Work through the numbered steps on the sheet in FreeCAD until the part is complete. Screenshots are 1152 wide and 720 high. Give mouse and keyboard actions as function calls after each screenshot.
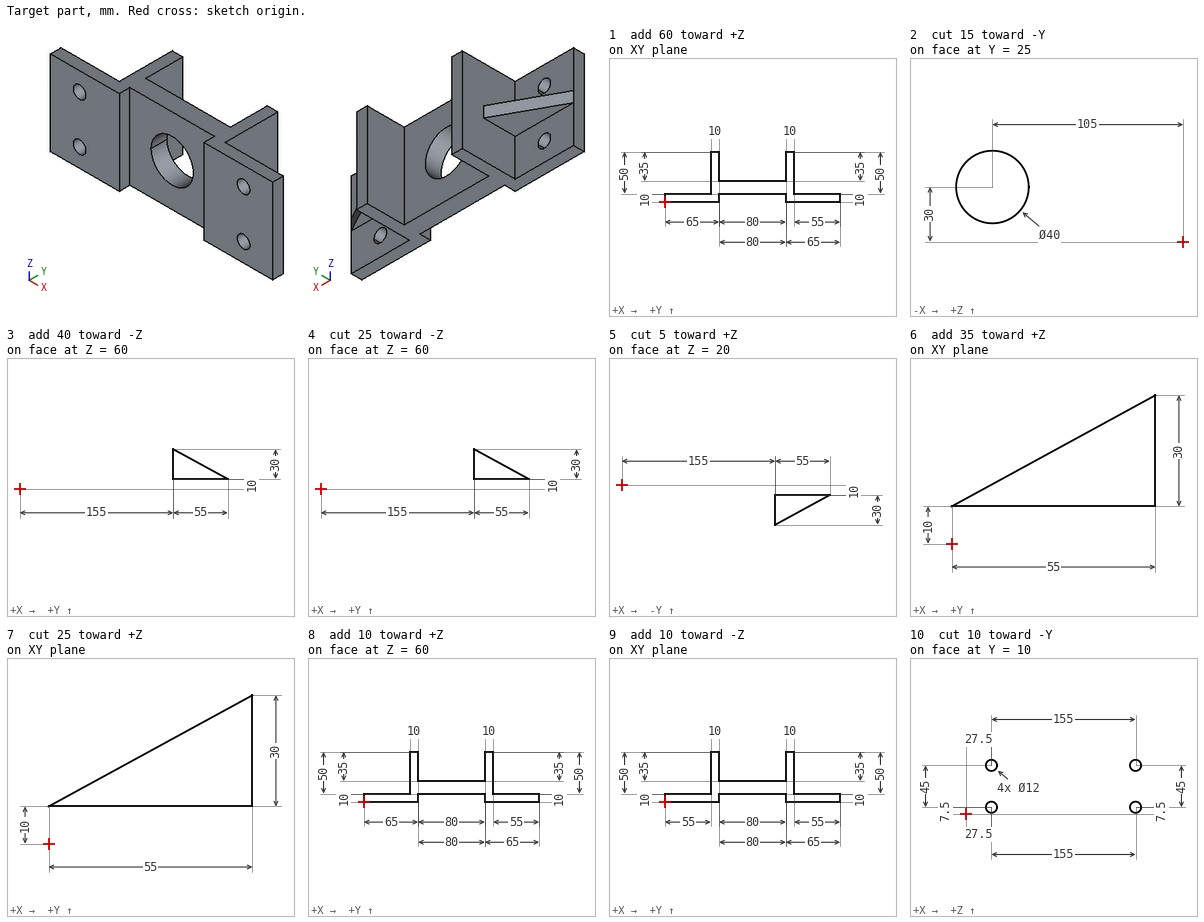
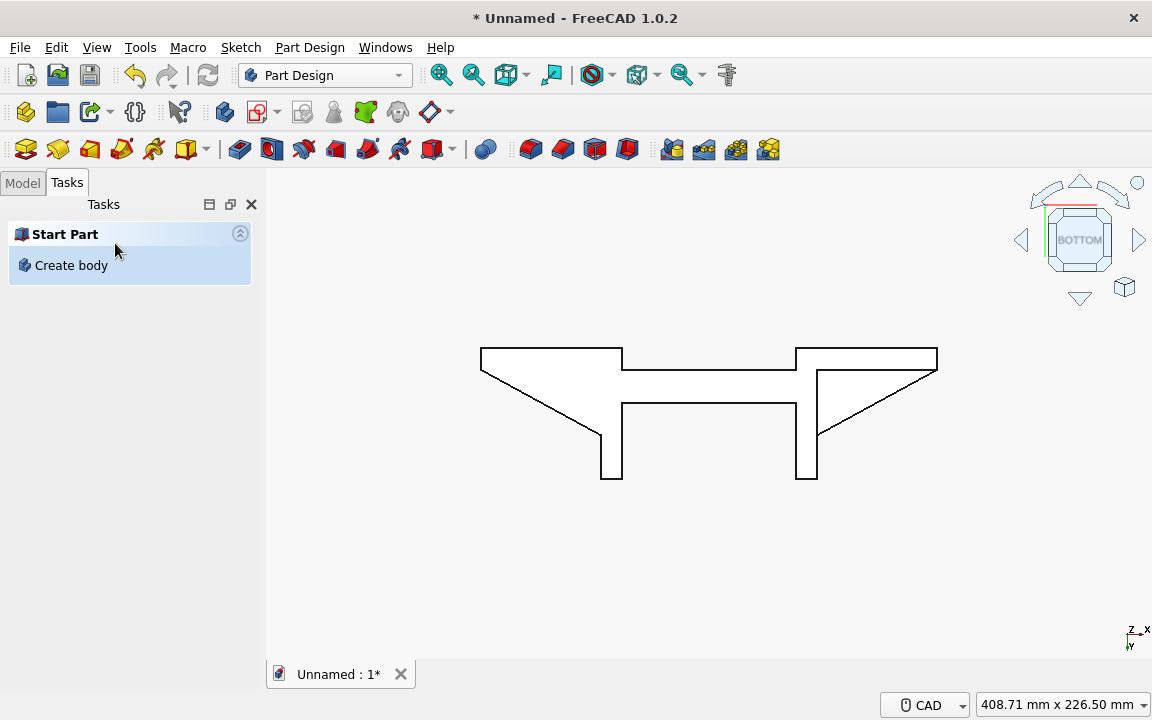
click(258, 112)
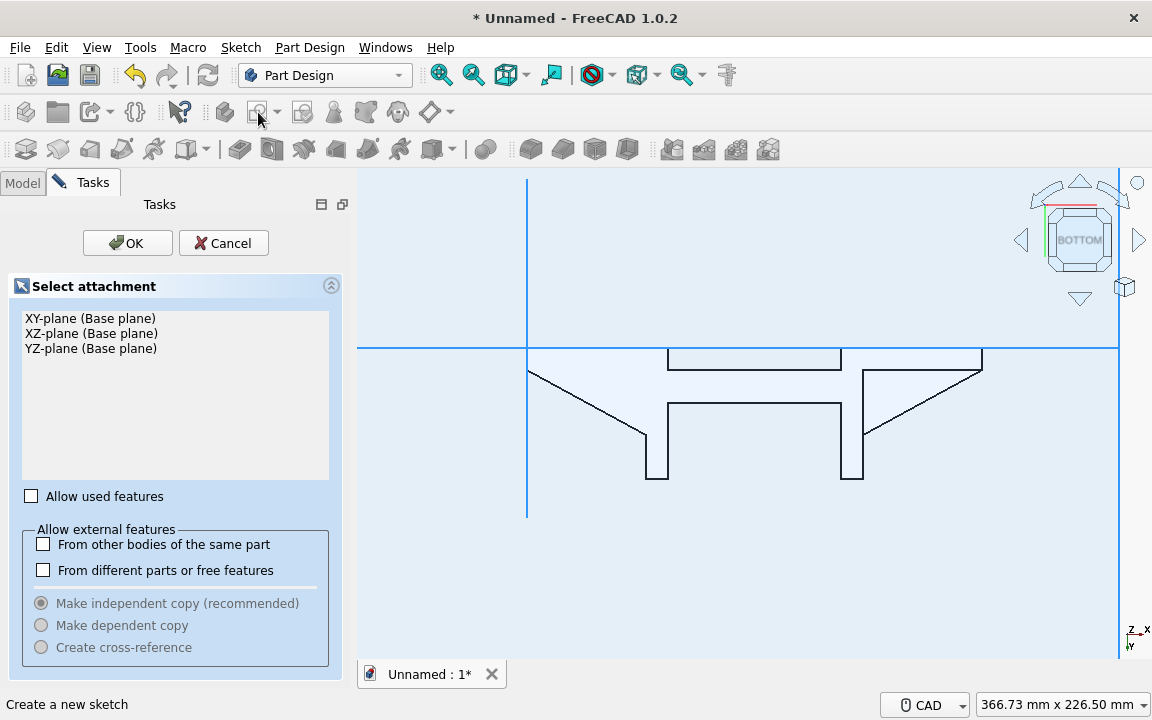
click(82, 318)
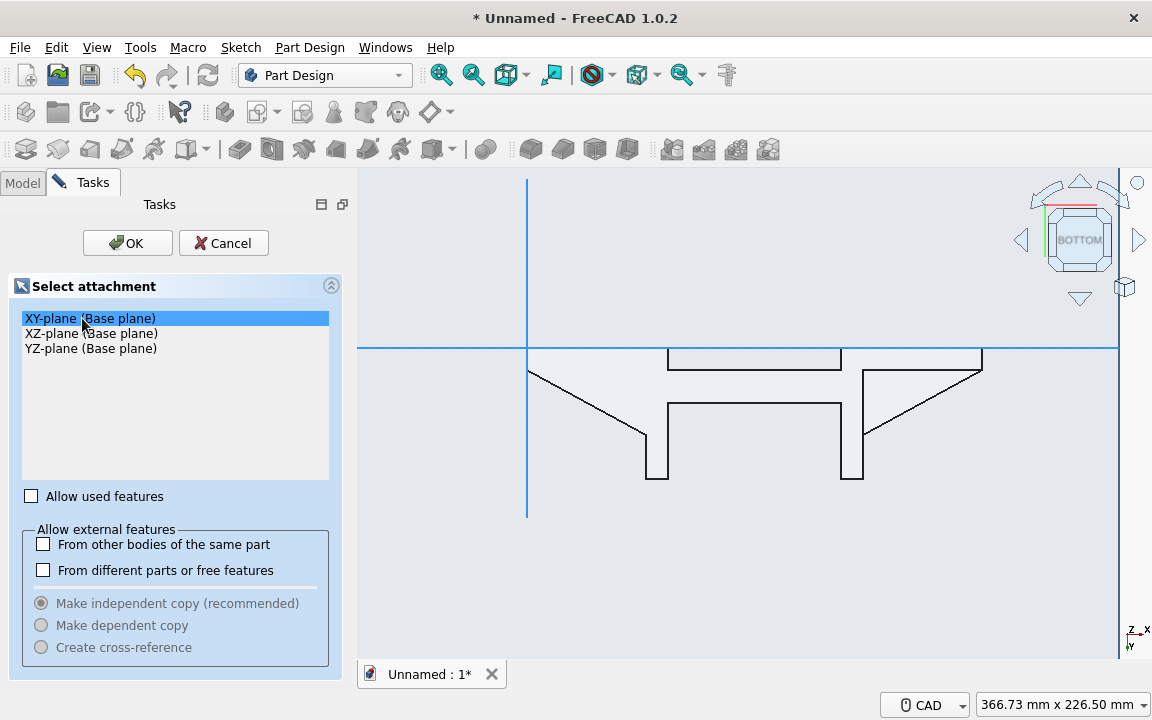
click(128, 243)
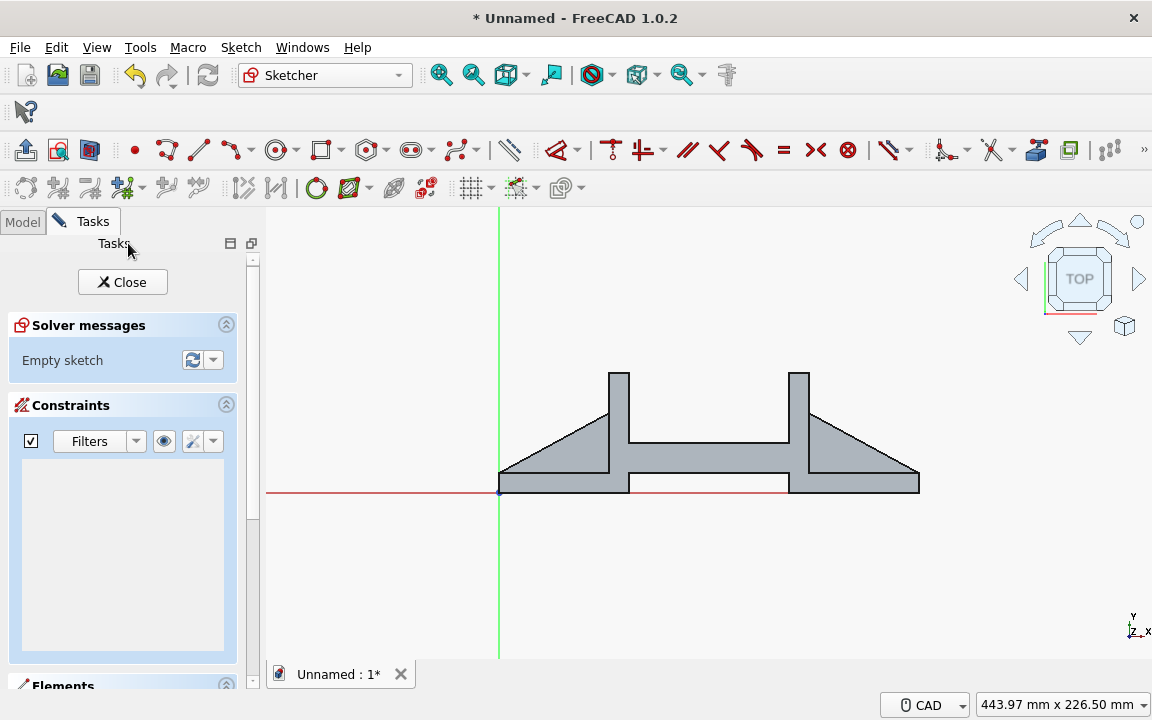
key(q)
key(s)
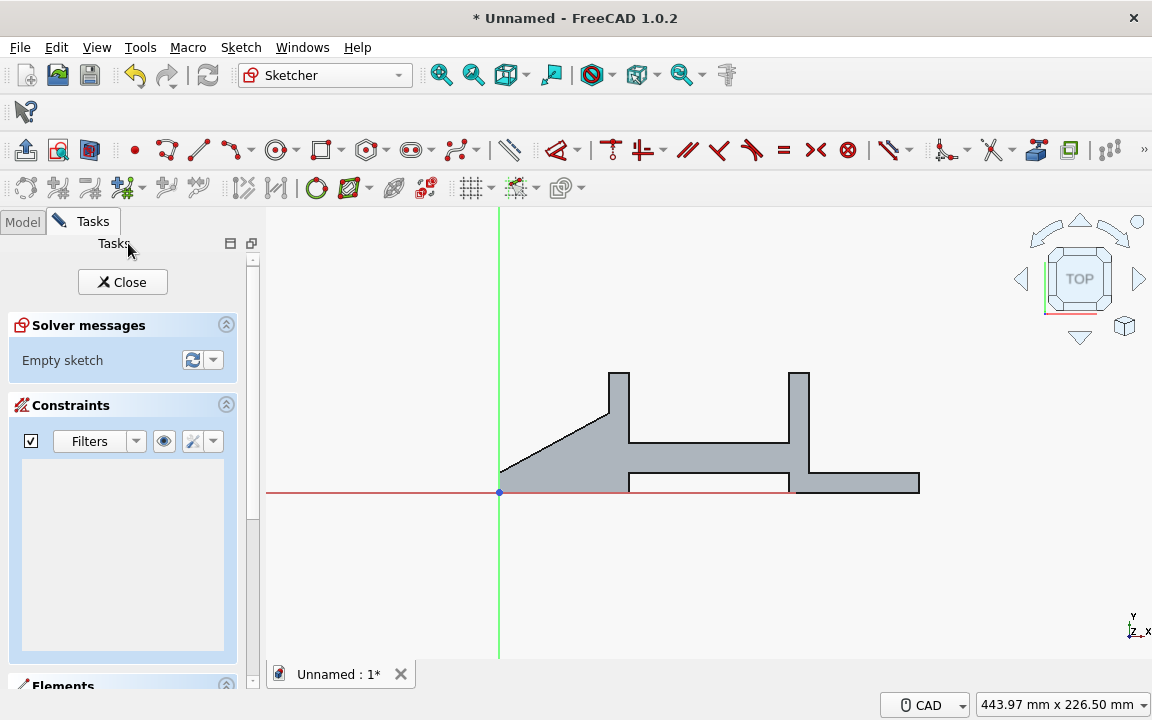
scroll(517, 462, up, 6)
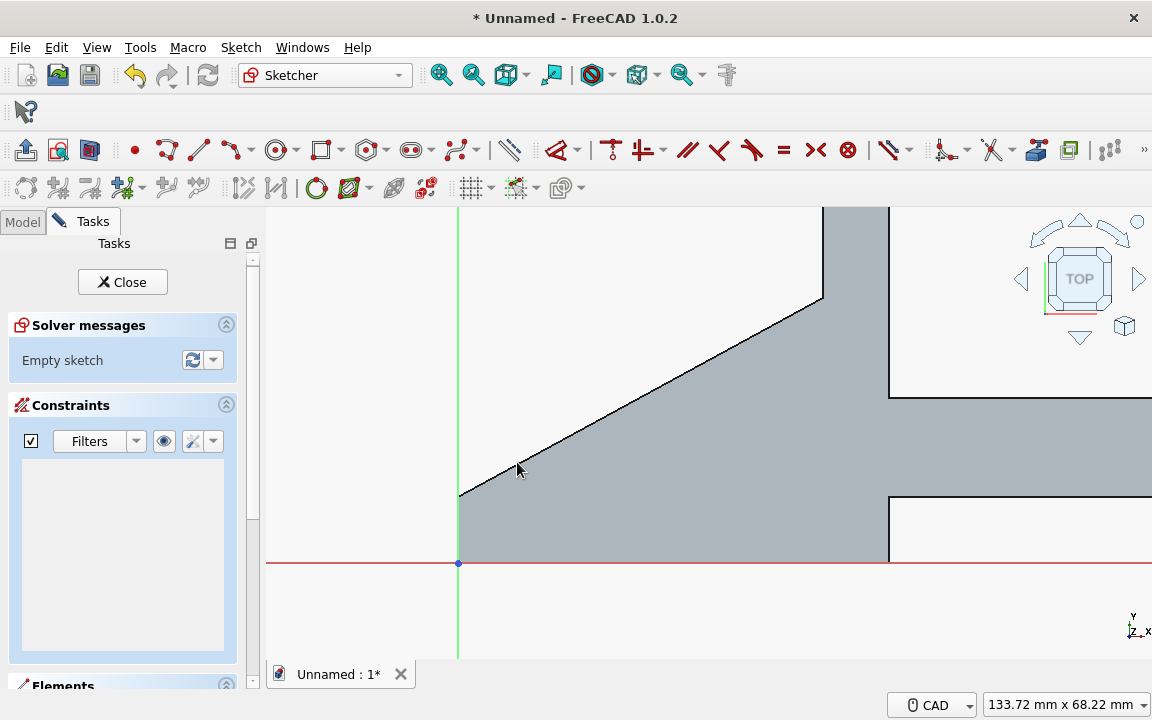
click(168, 150)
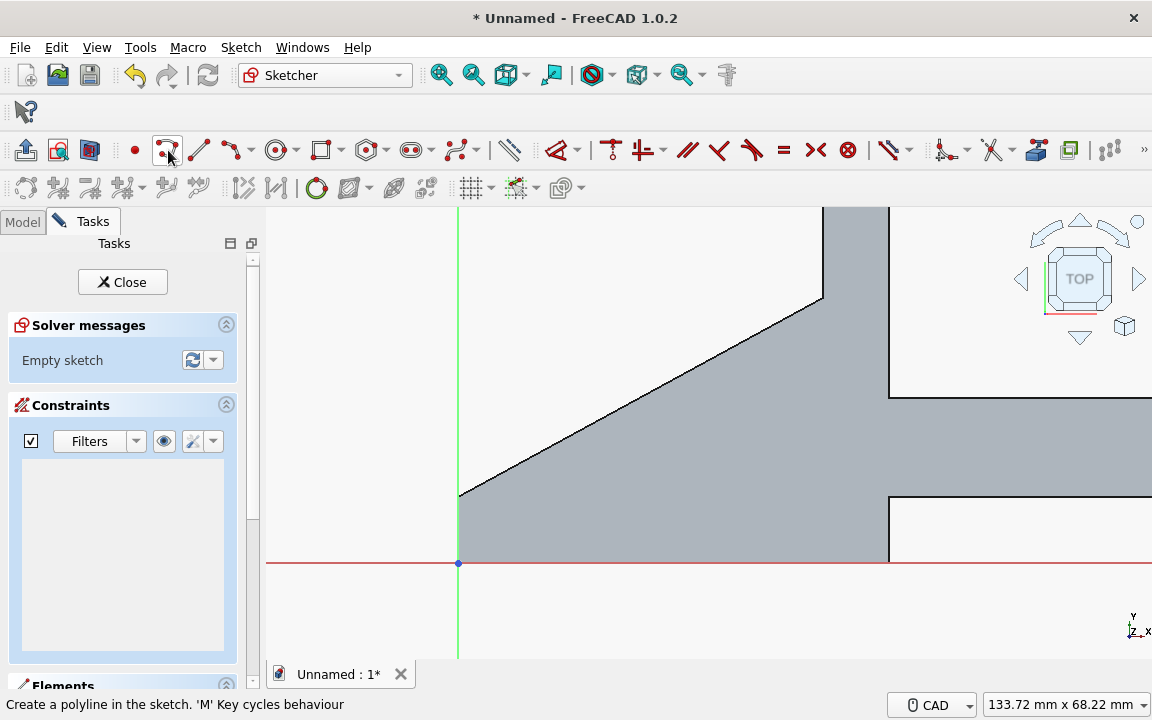
click(458, 497)
click(823, 298)
click(823, 497)
click(458, 498)
key(Escape)
key(Escape)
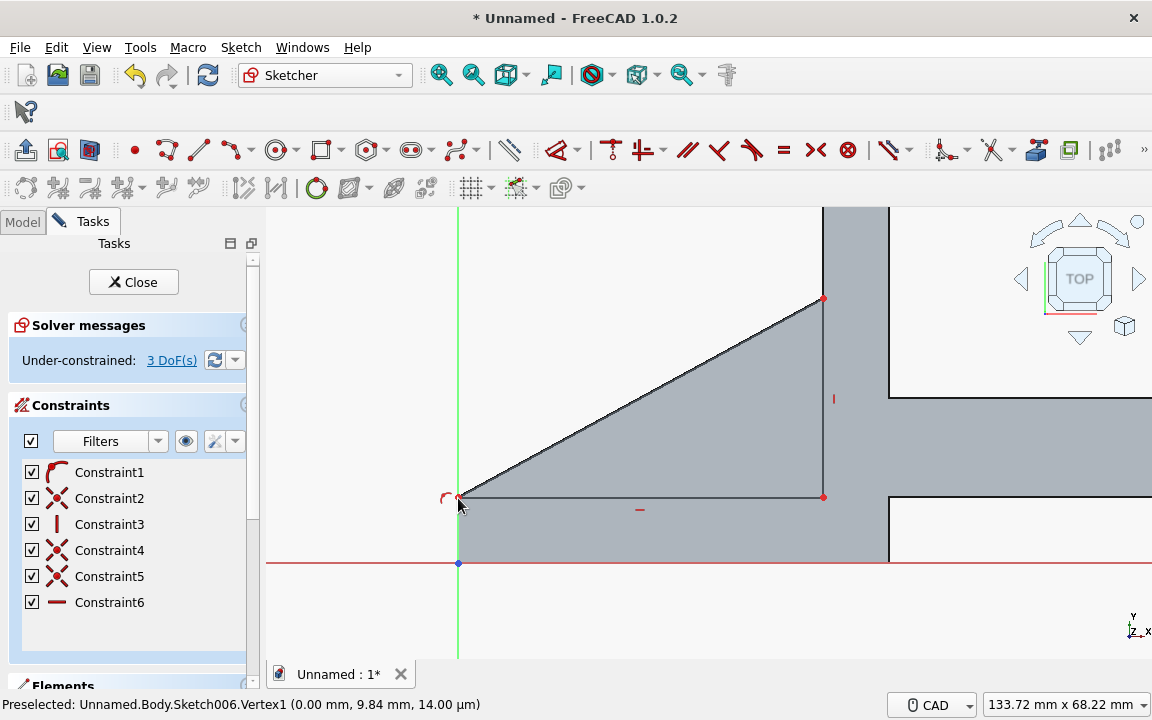
key(d)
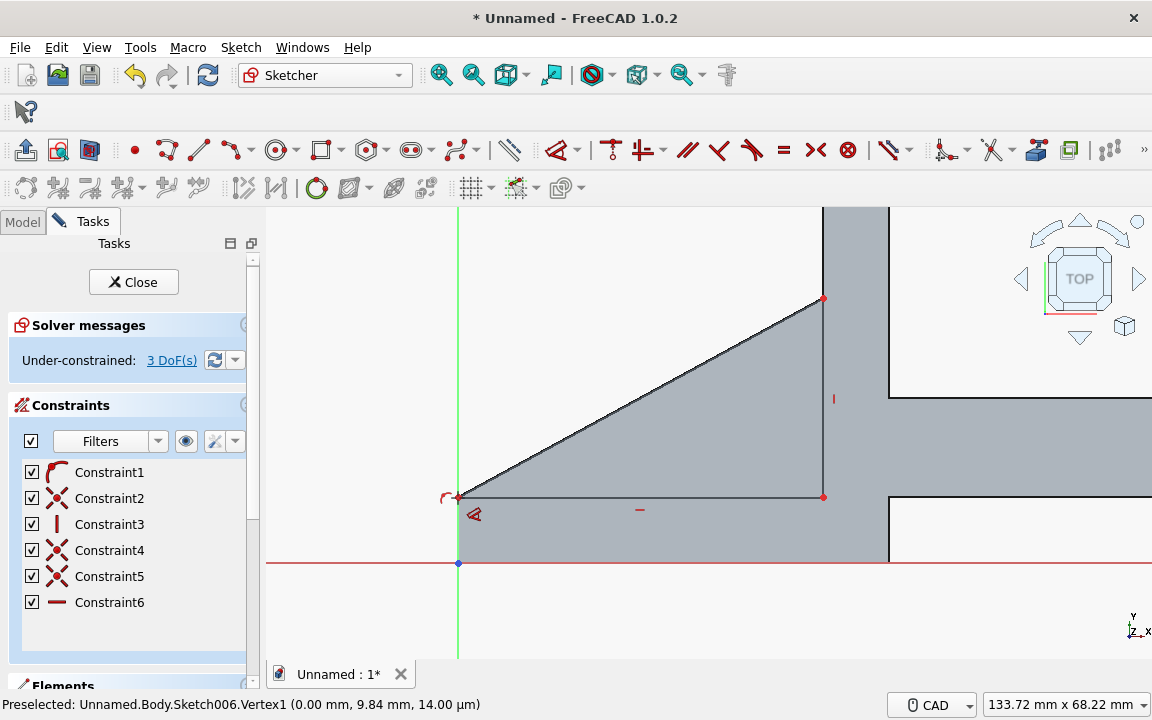
click(823, 359)
click(857, 399)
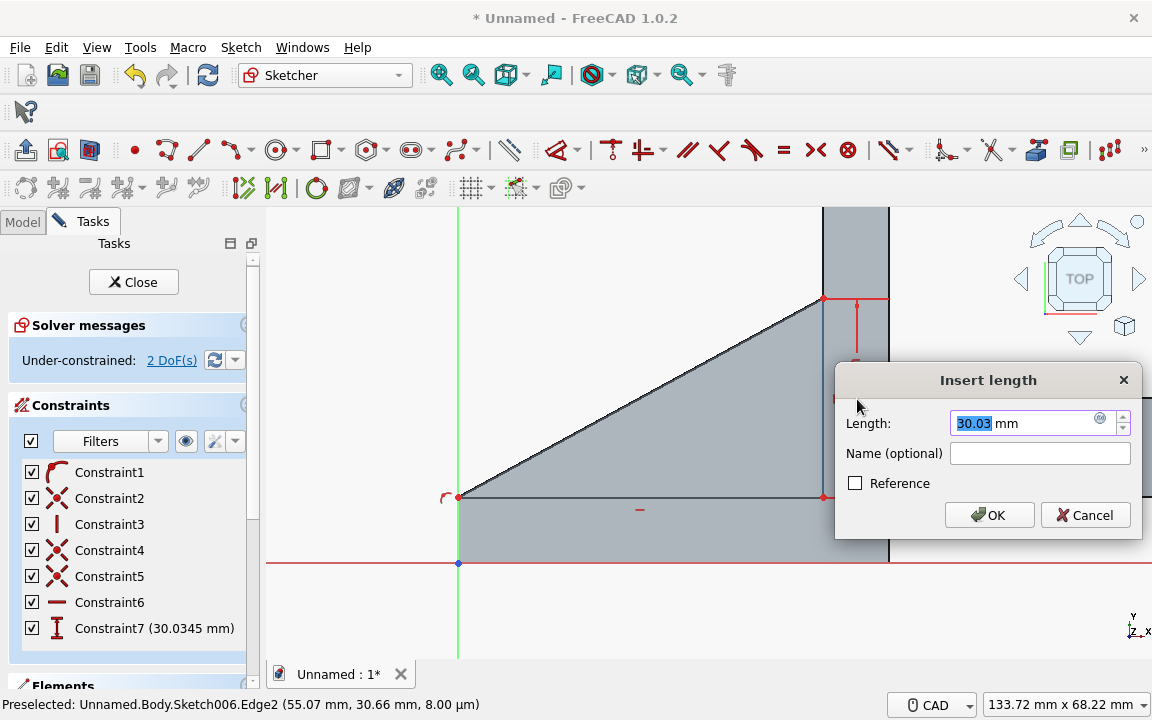
text(30)
key(Return)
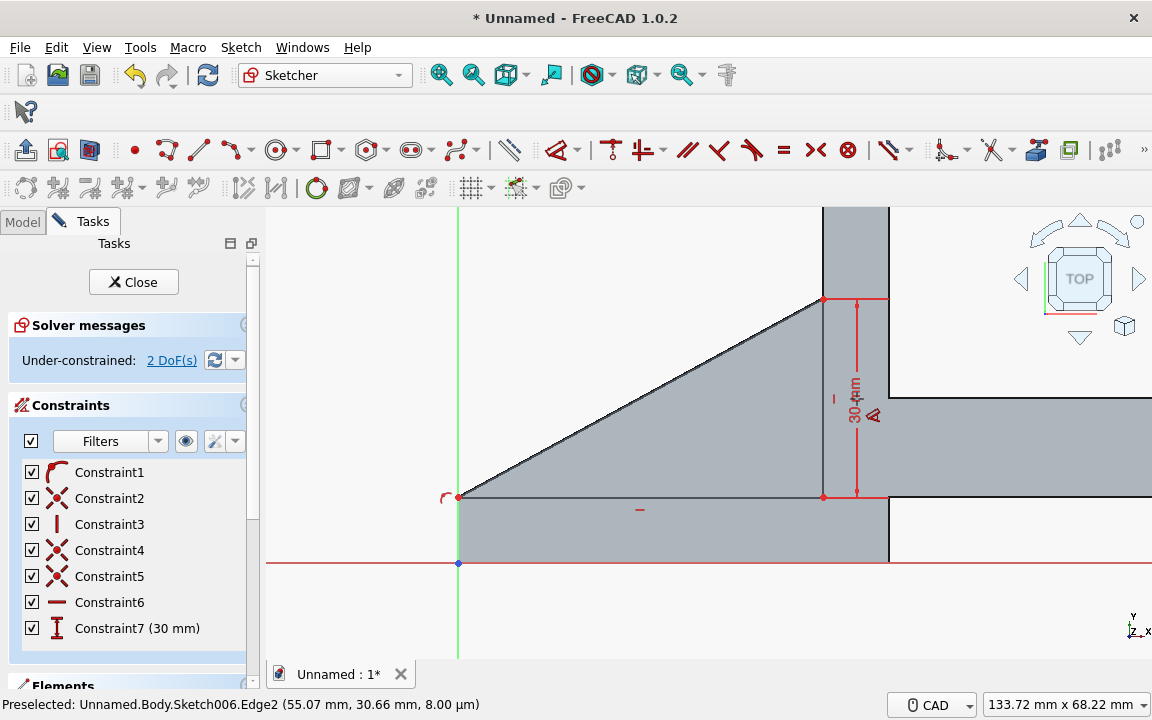
click(714, 498)
click(641, 532)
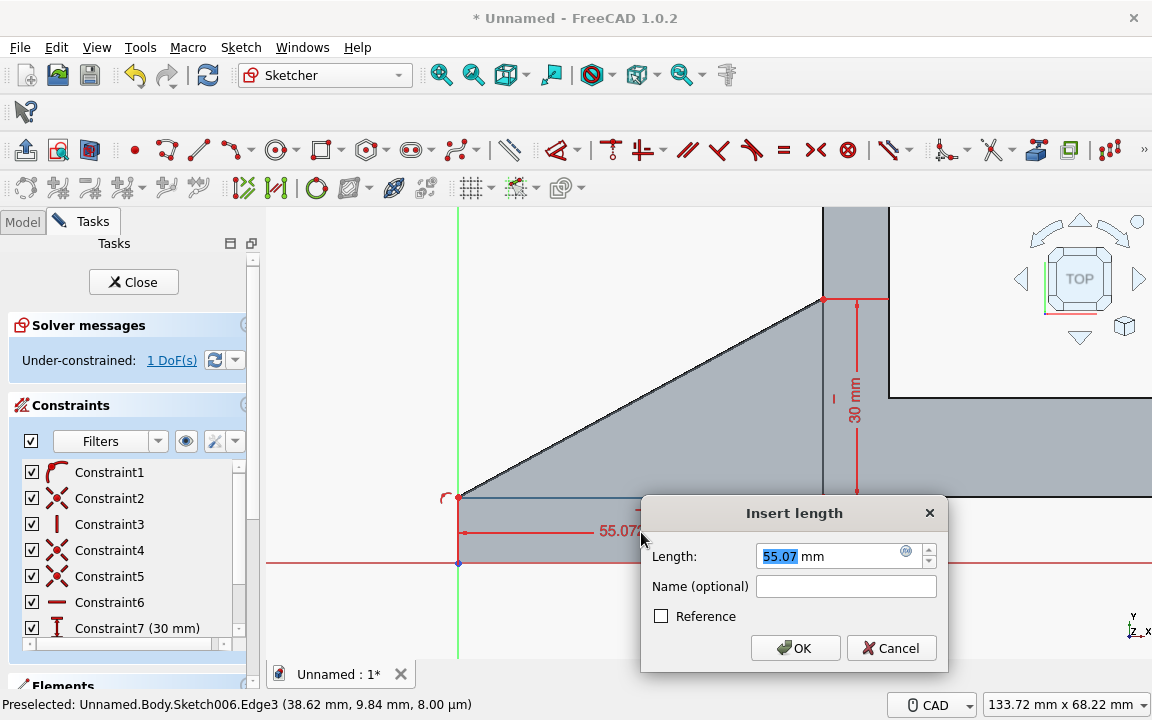
text(55)
key(Return)